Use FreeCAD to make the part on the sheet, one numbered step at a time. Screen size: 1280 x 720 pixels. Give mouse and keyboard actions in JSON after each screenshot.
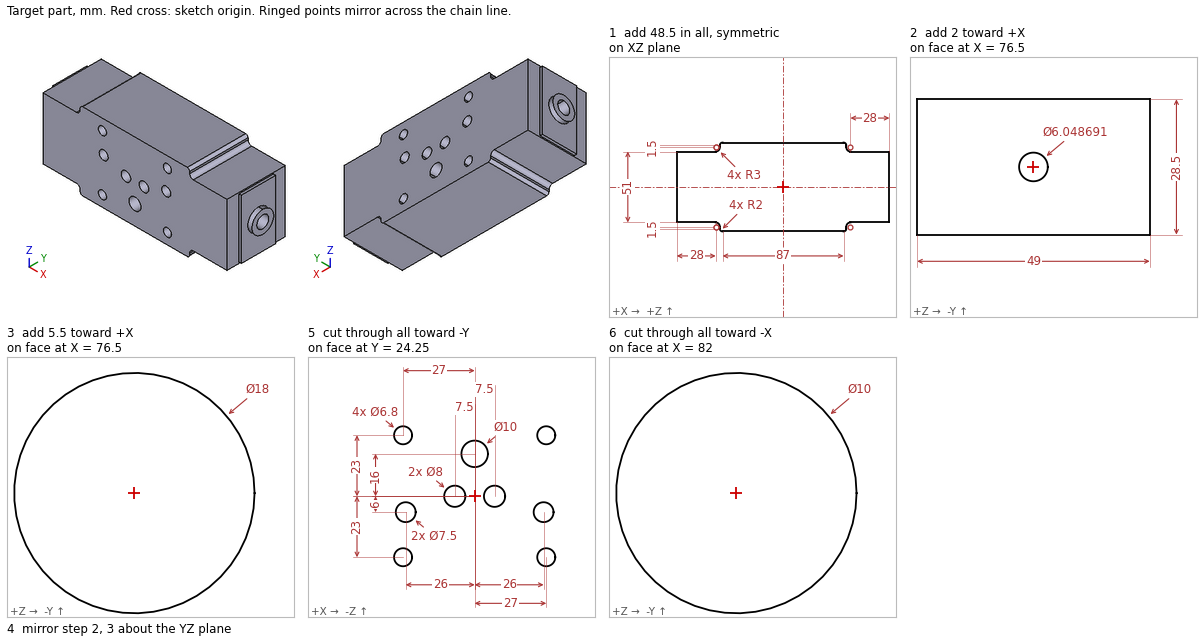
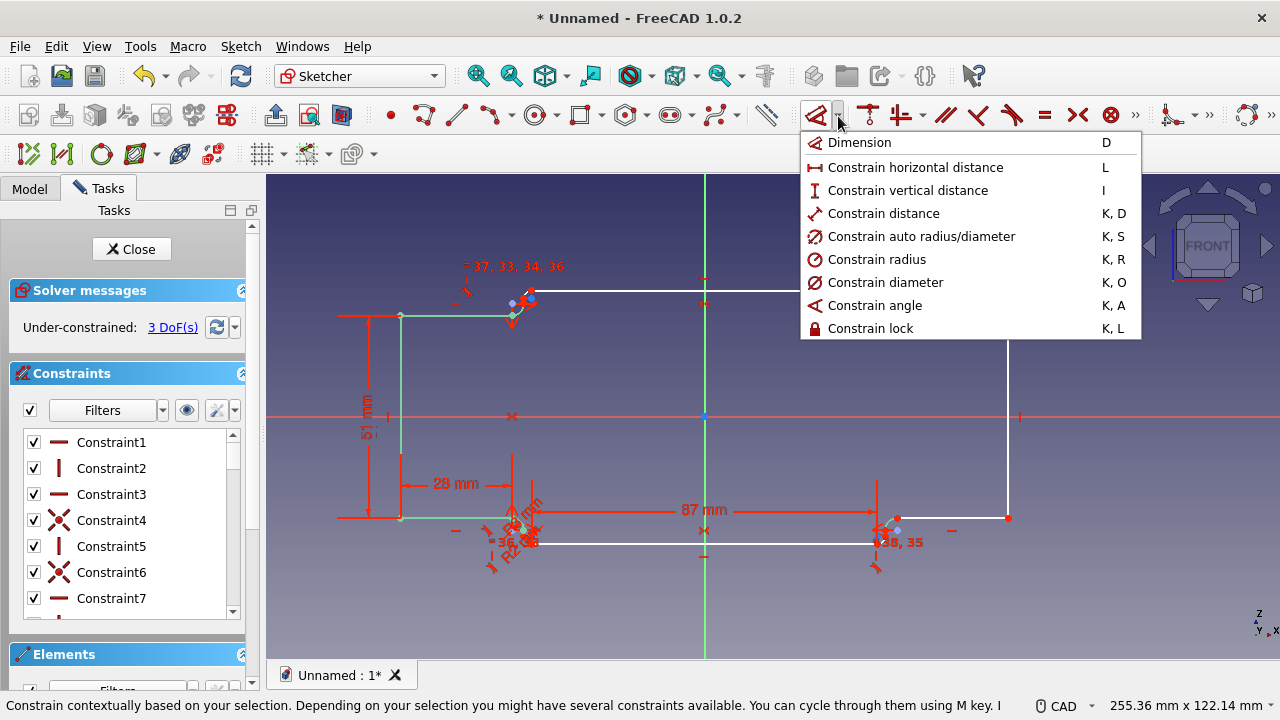
{"action": "left_click", "coordinate": [971, 168]}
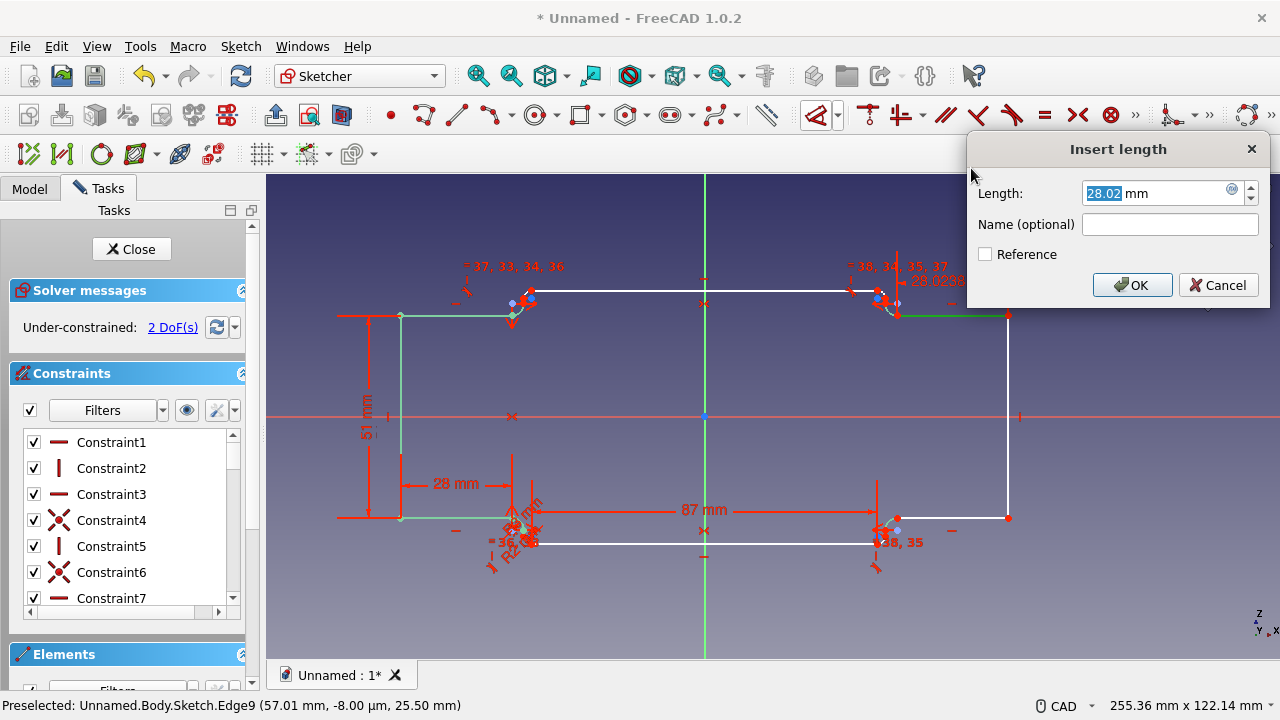
{"action": "type", "text": "28"}
{"action": "key", "text": "Return"}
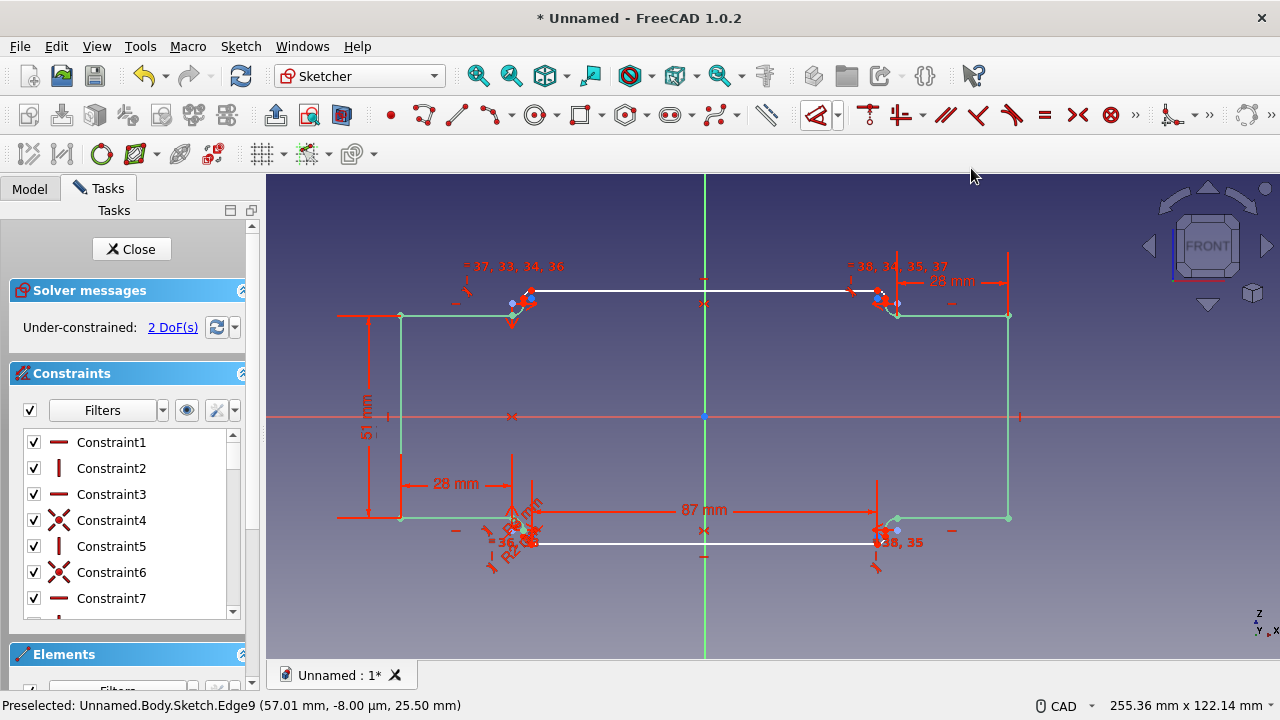
{"action": "scroll", "coordinate": [524, 533], "scroll_direction": "up", "scroll_amount": 10}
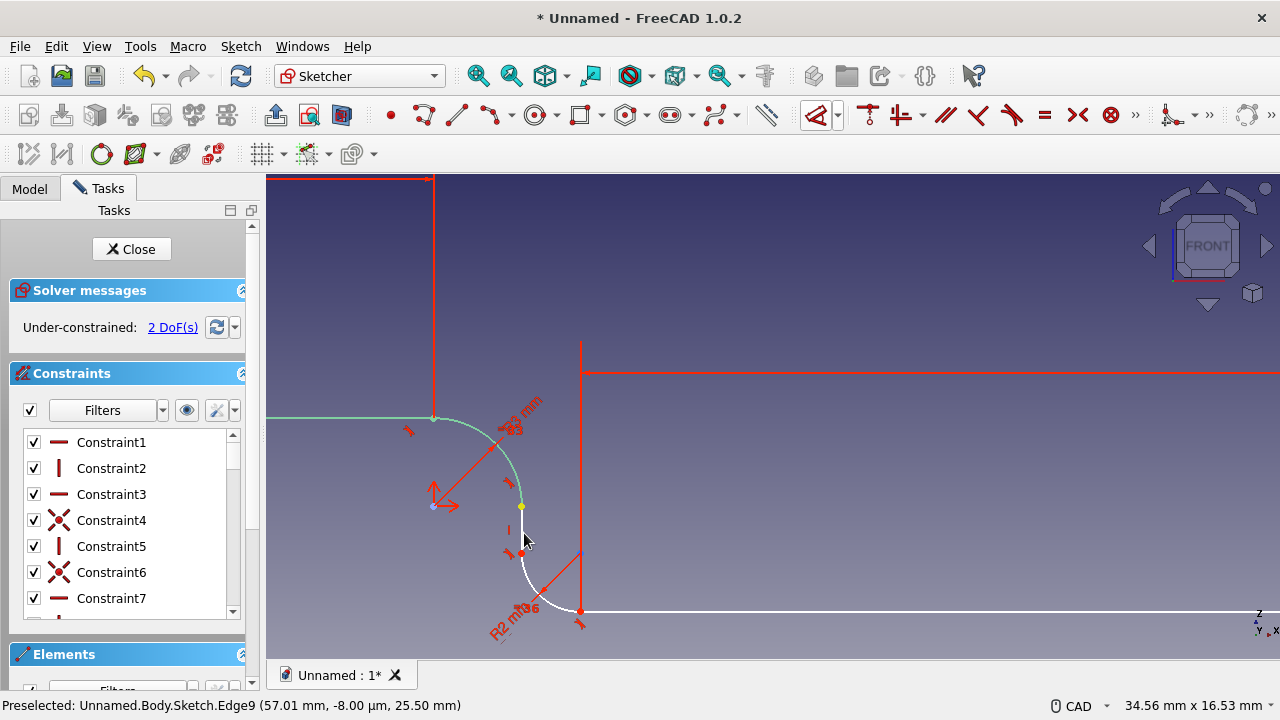
{"action": "left_click", "coordinate": [522, 530]}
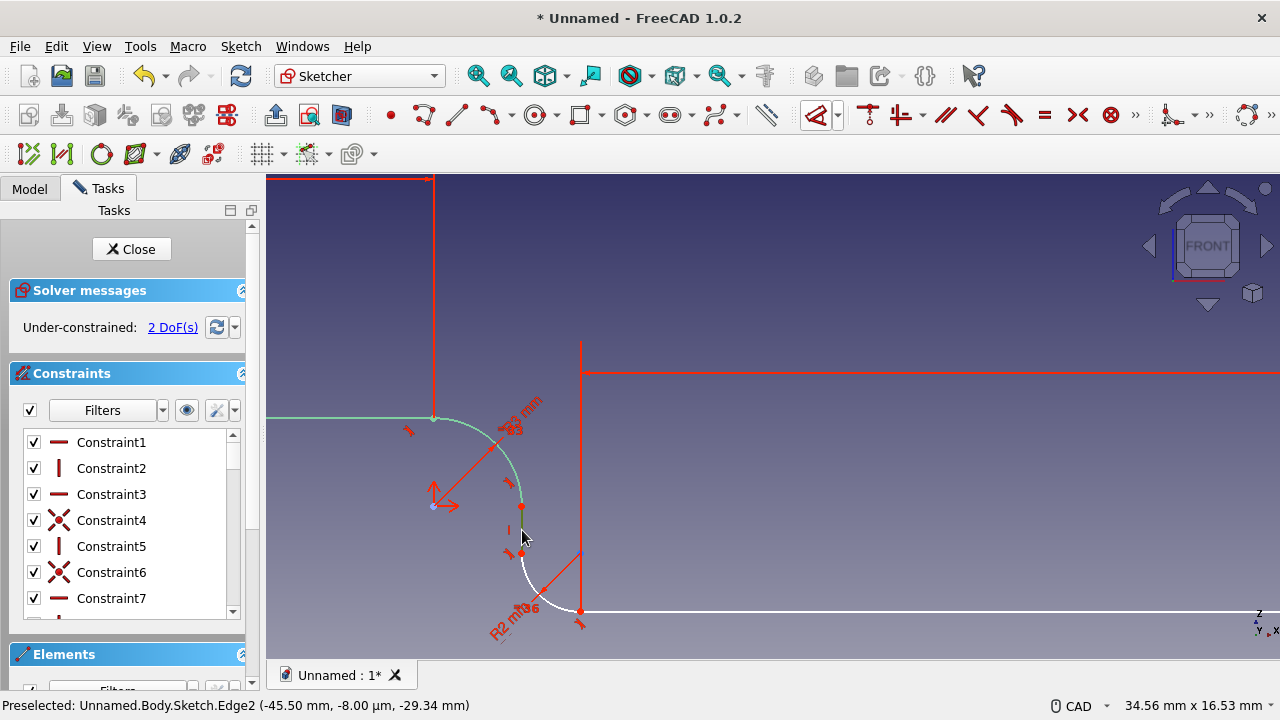
{"action": "left_click", "coordinate": [838, 116]}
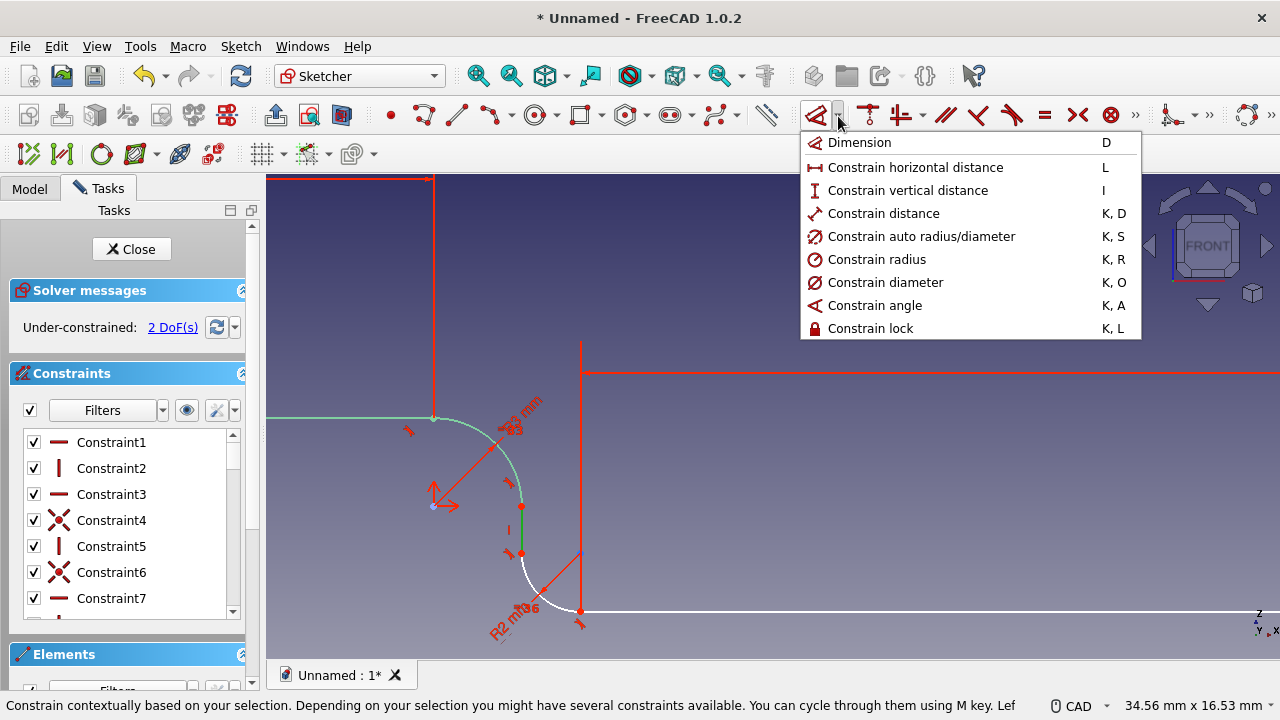
{"action": "left_click", "coordinate": [971, 190]}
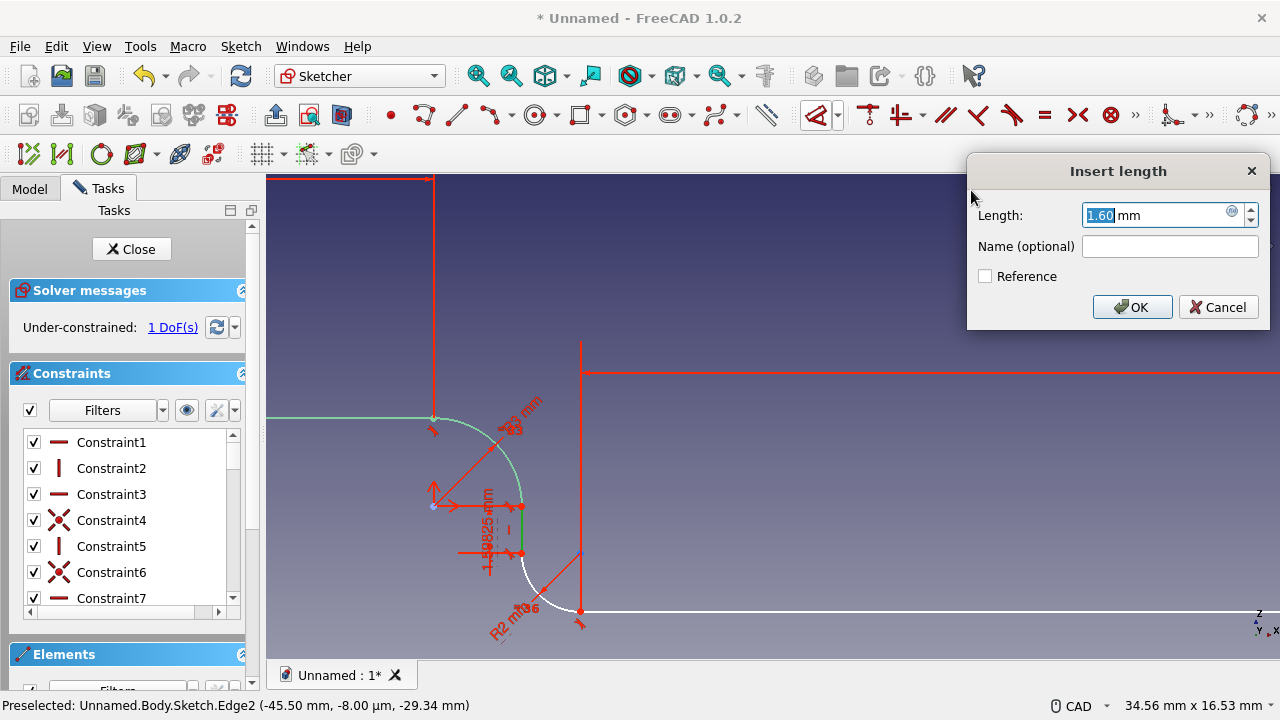
{"action": "type", "text": "1.5"}
{"action": "key", "text": "Return"}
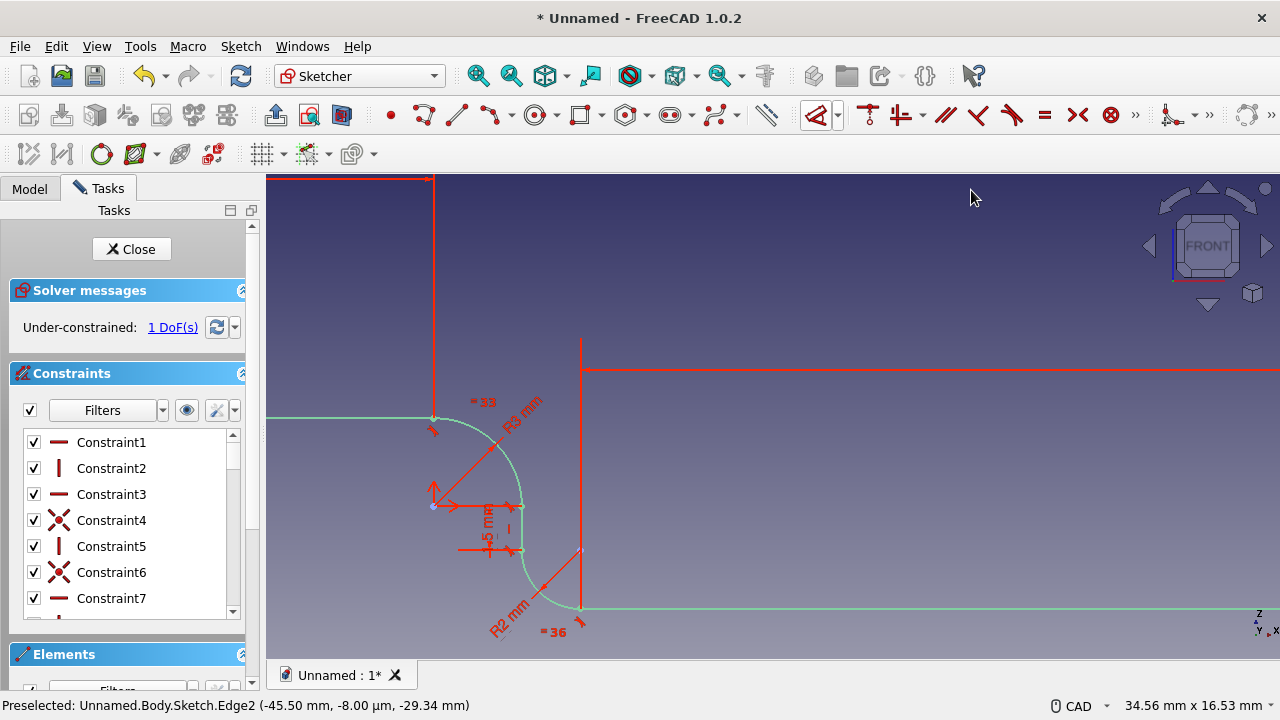
{"action": "scroll", "coordinate": [524, 533], "scroll_direction": "down", "scroll_amount": 10}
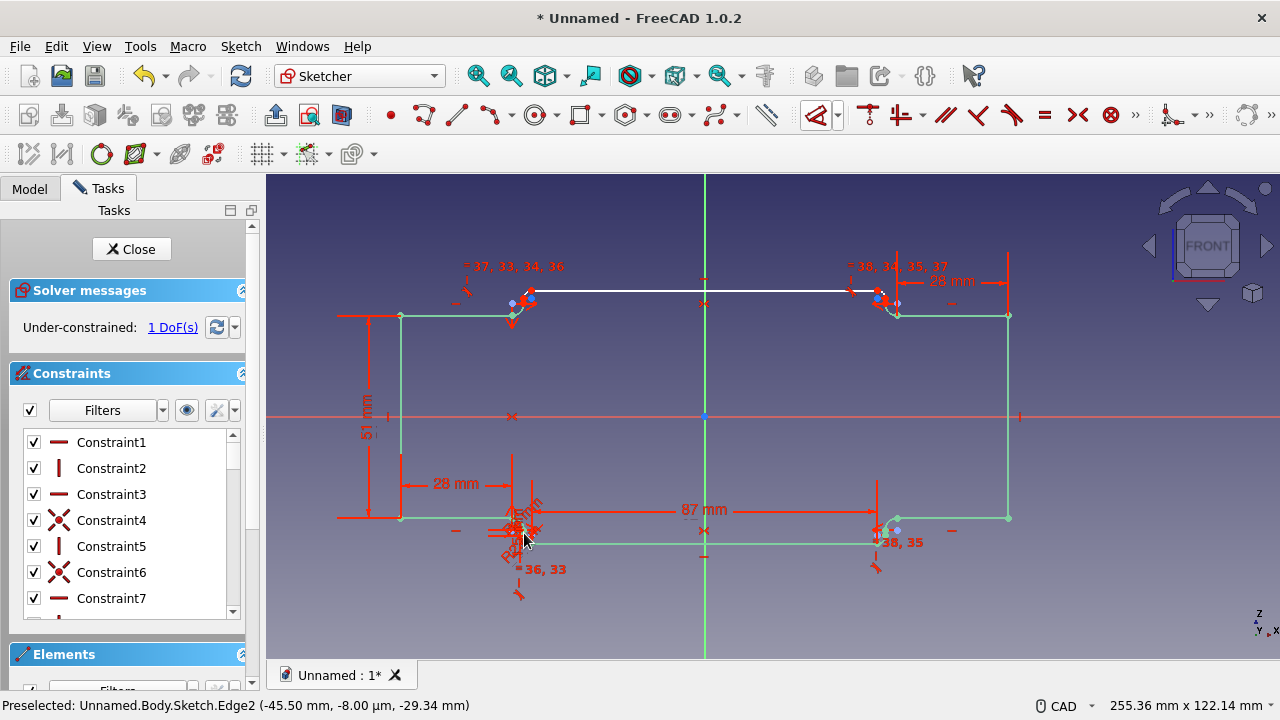
{"action": "scroll", "coordinate": [524, 302], "scroll_direction": "up", "scroll_amount": 11}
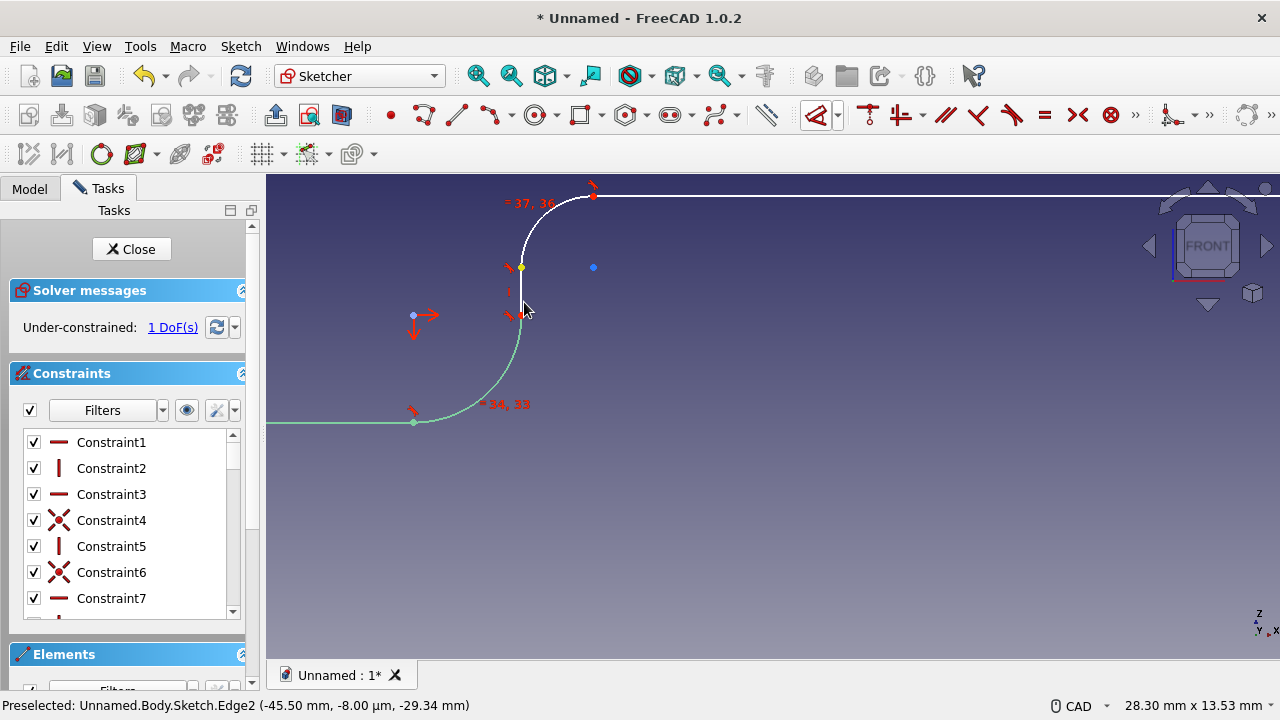
{"action": "left_click", "coordinate": [521, 301]}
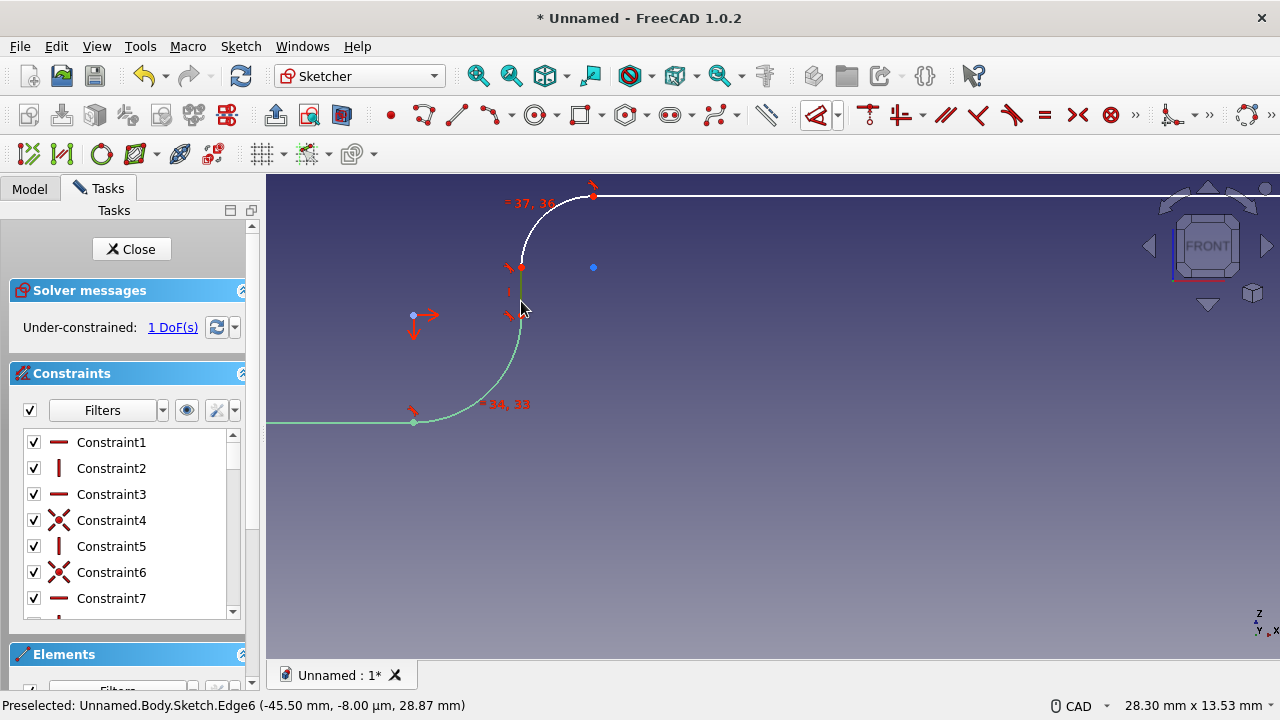
{"action": "left_click", "coordinate": [838, 116]}